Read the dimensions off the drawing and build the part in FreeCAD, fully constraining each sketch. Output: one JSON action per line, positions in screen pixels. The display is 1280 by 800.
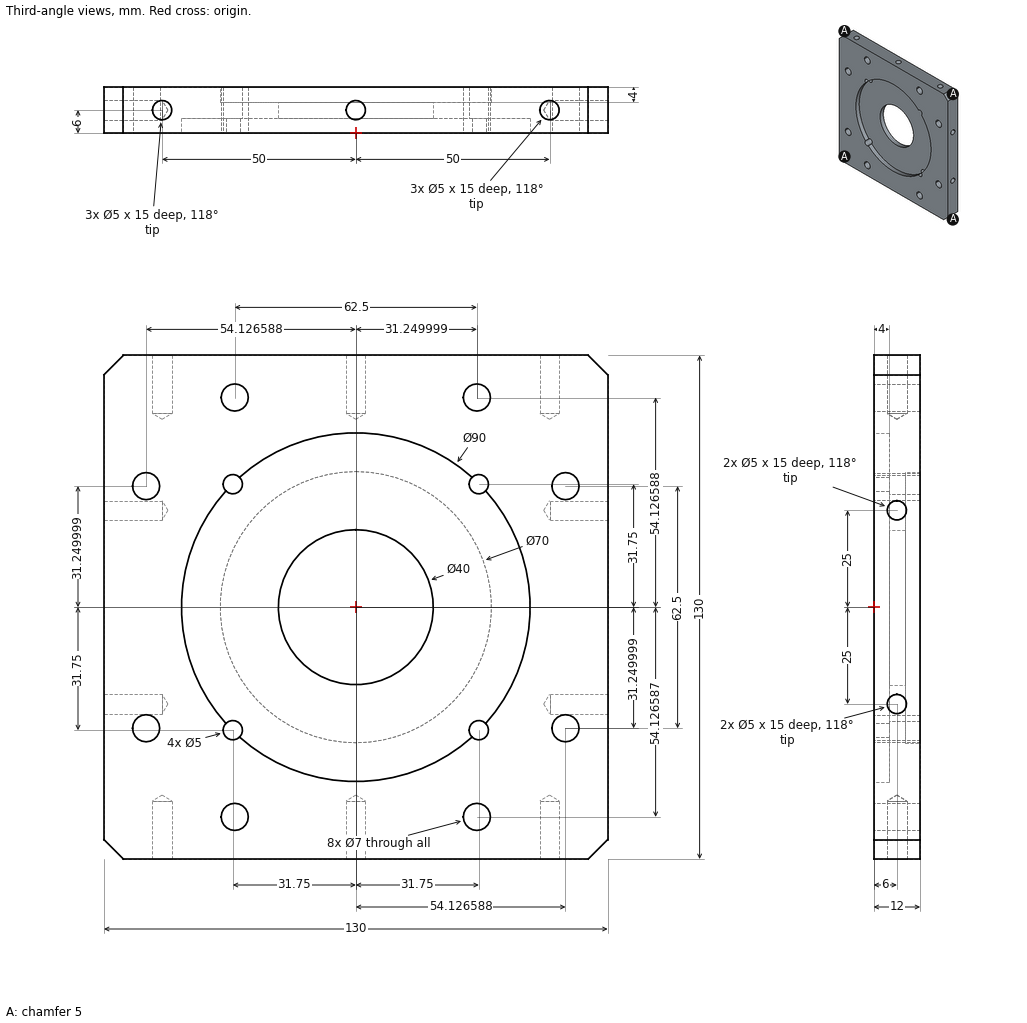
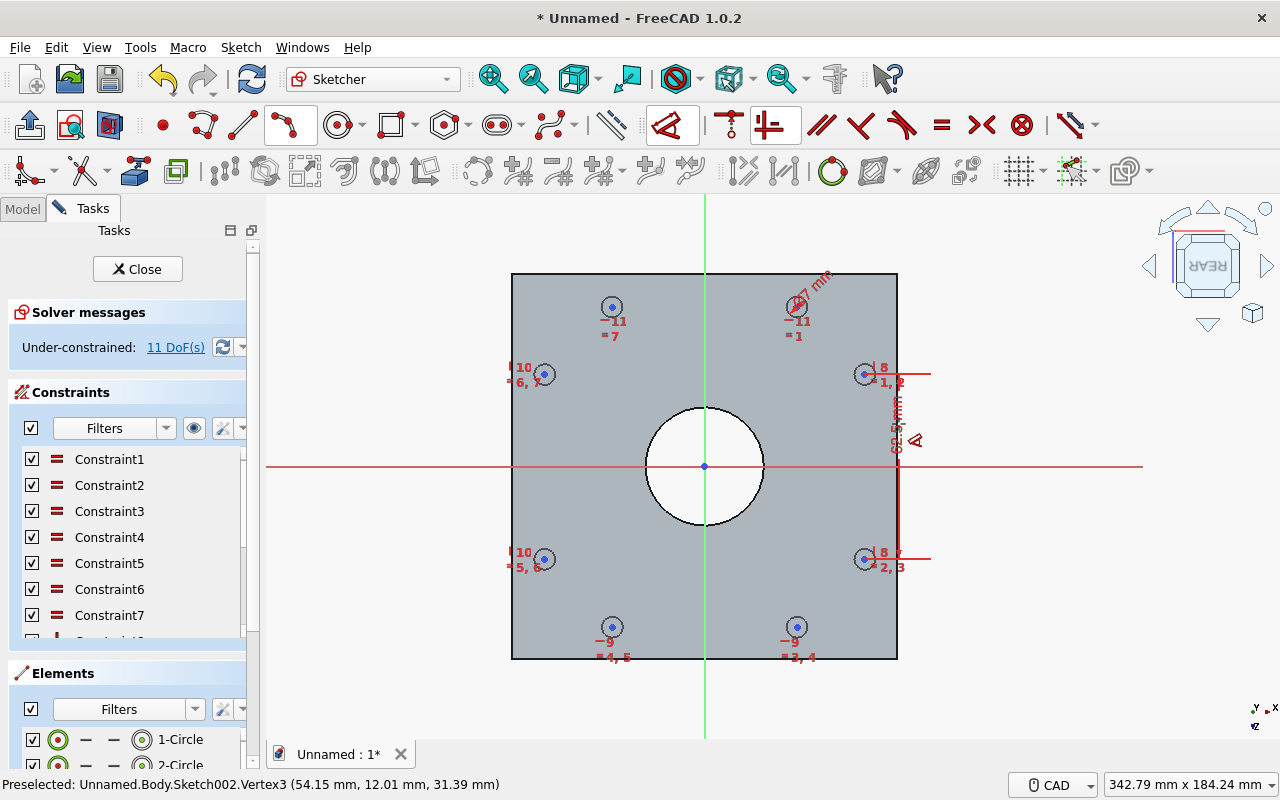
{"action": "left_click", "coordinate": [797, 627]}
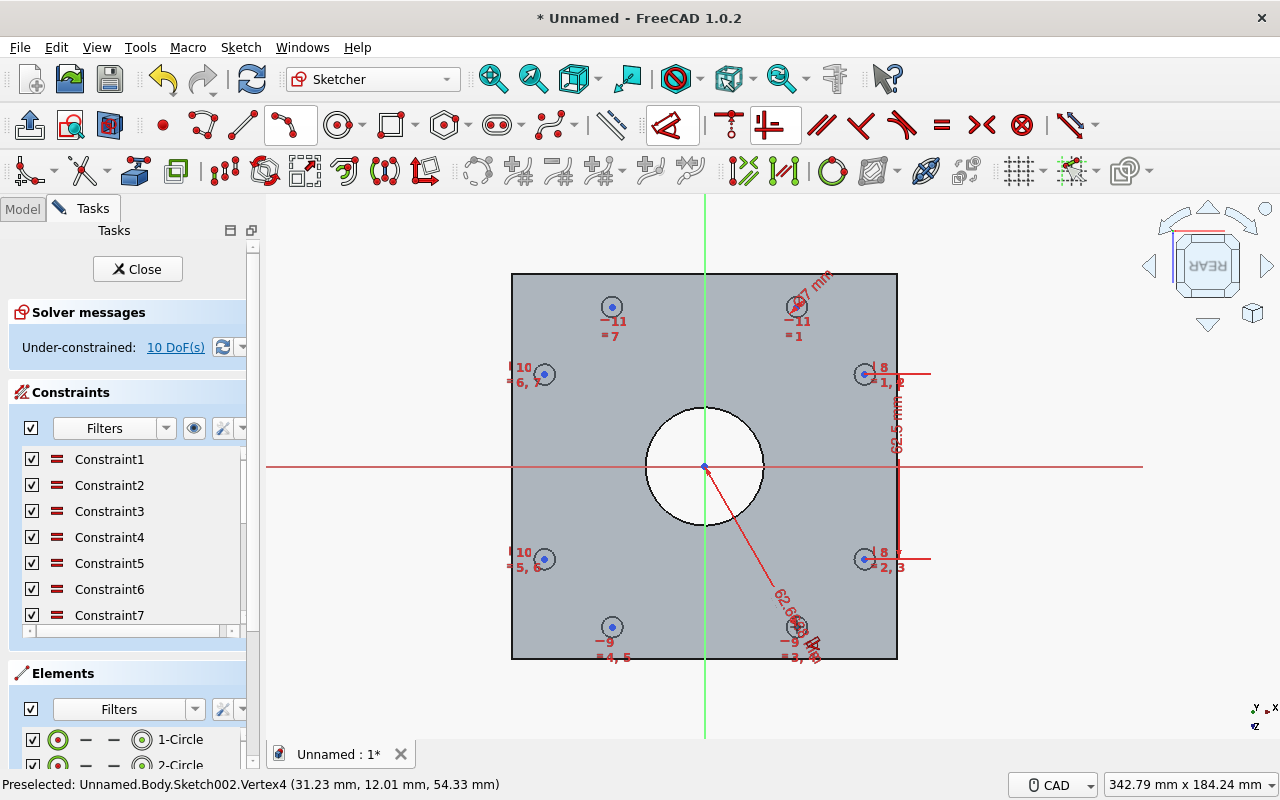
{"action": "left_click", "coordinate": [612, 627]}
{"action": "left_click", "coordinate": [662, 661]}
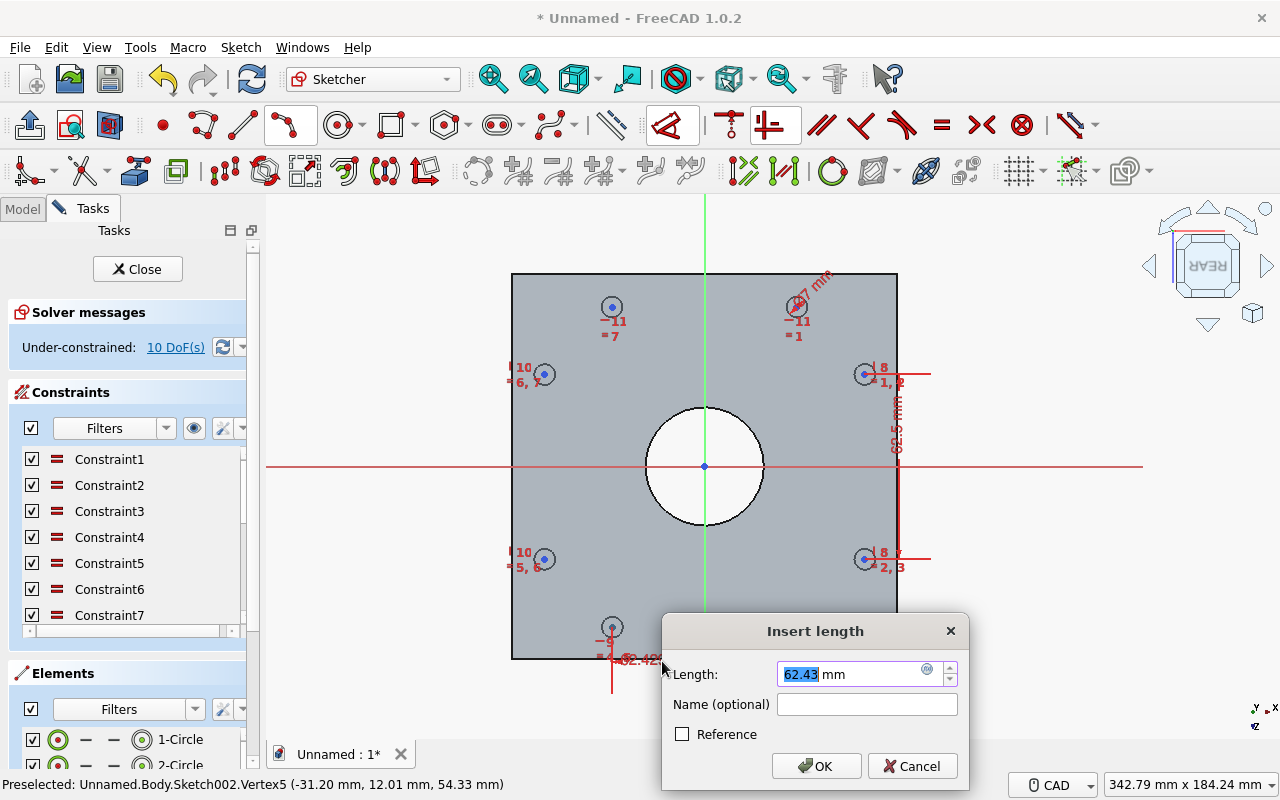
{"action": "type", "text": "62.5"}
{"action": "key", "text": "Return"}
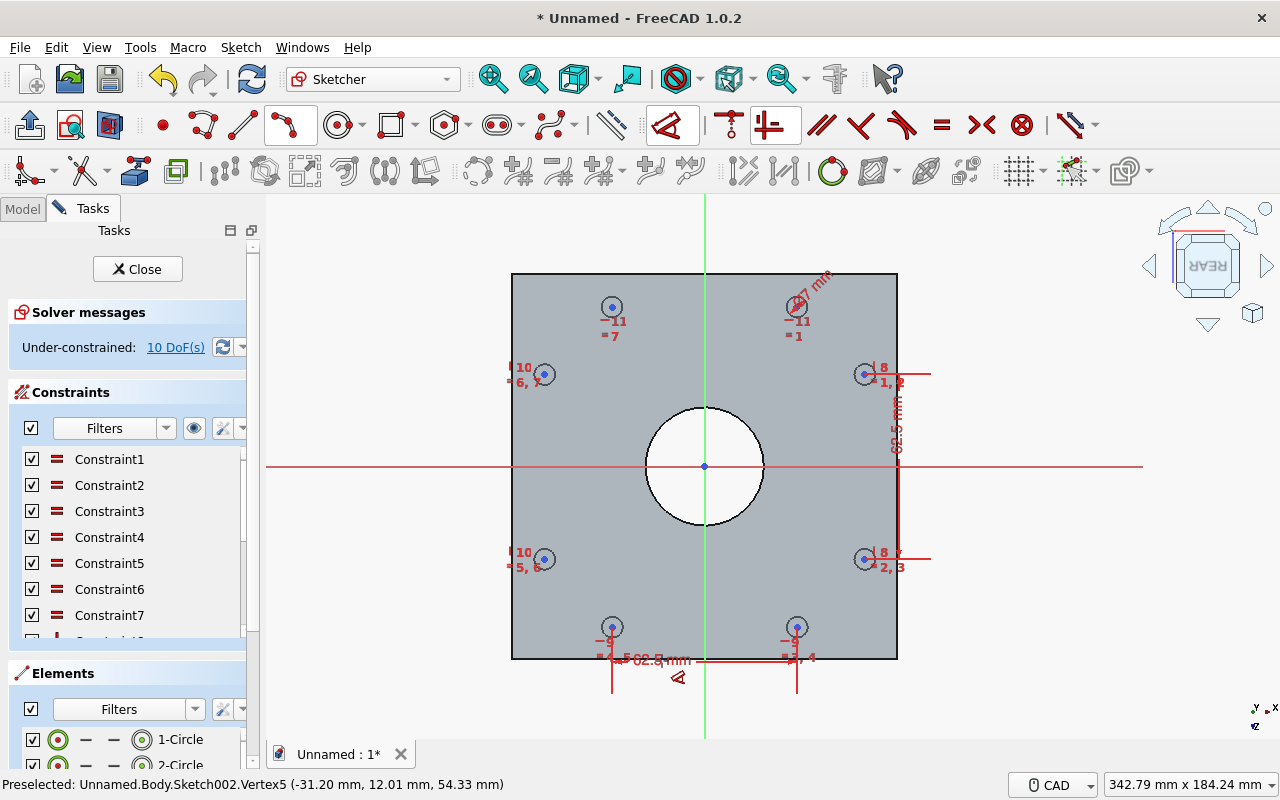
{"action": "left_click", "coordinate": [545, 559]}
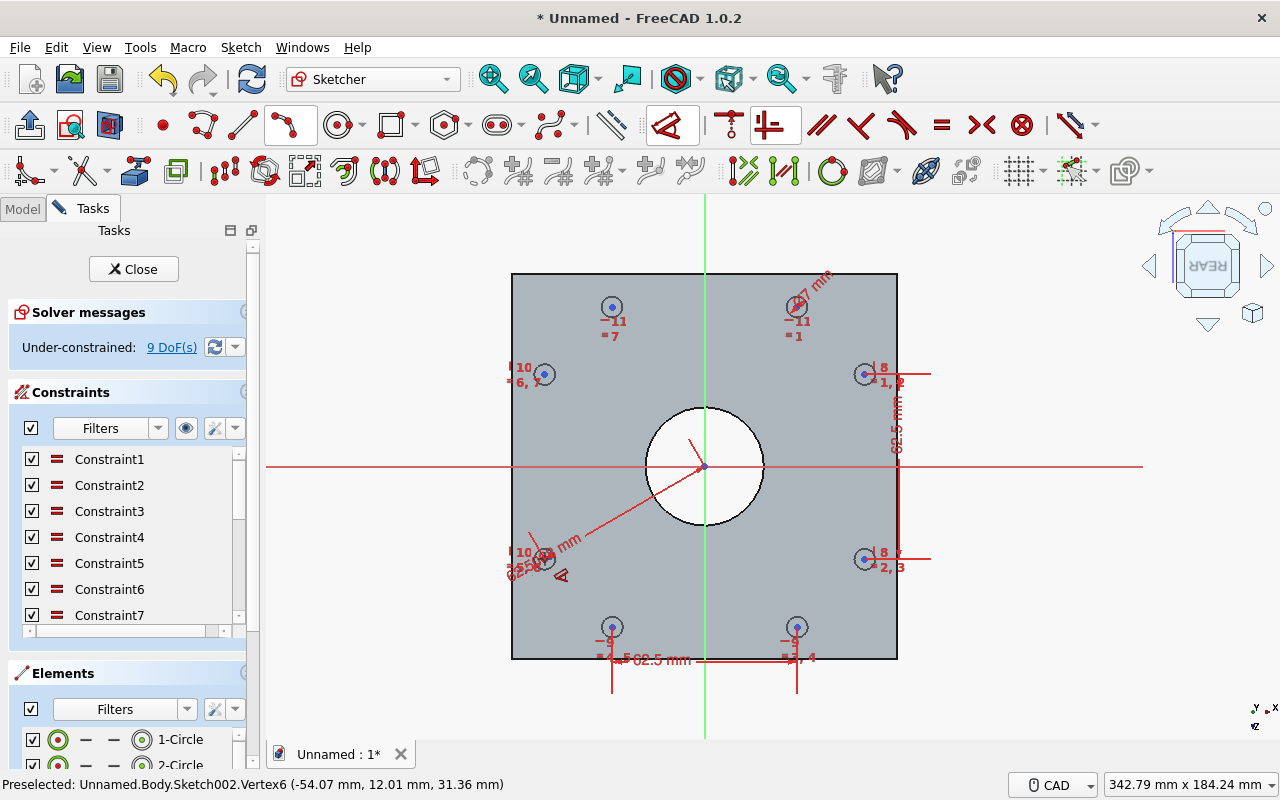
{"action": "left_click", "coordinate": [545, 375]}
{"action": "left_click", "coordinate": [511, 424]}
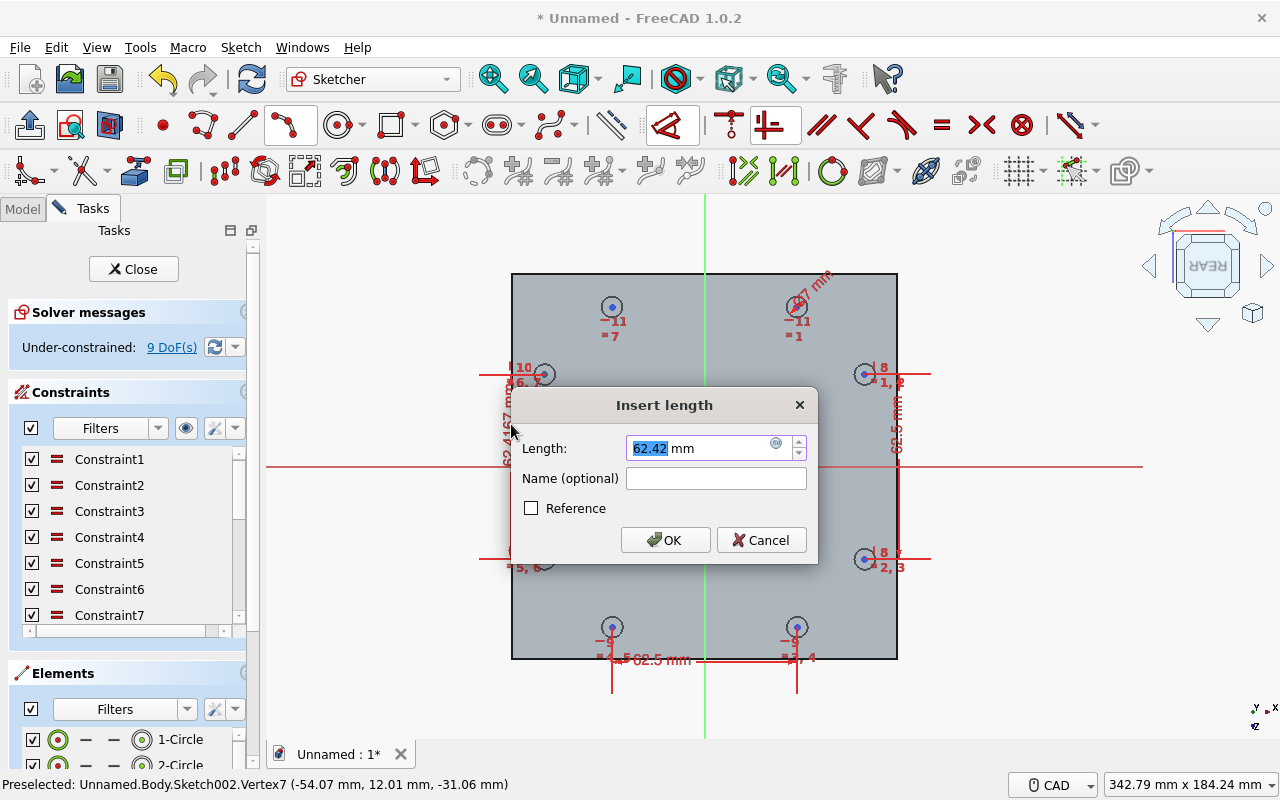
{"action": "type", "text": "62.5"}
{"action": "key", "text": "Return"}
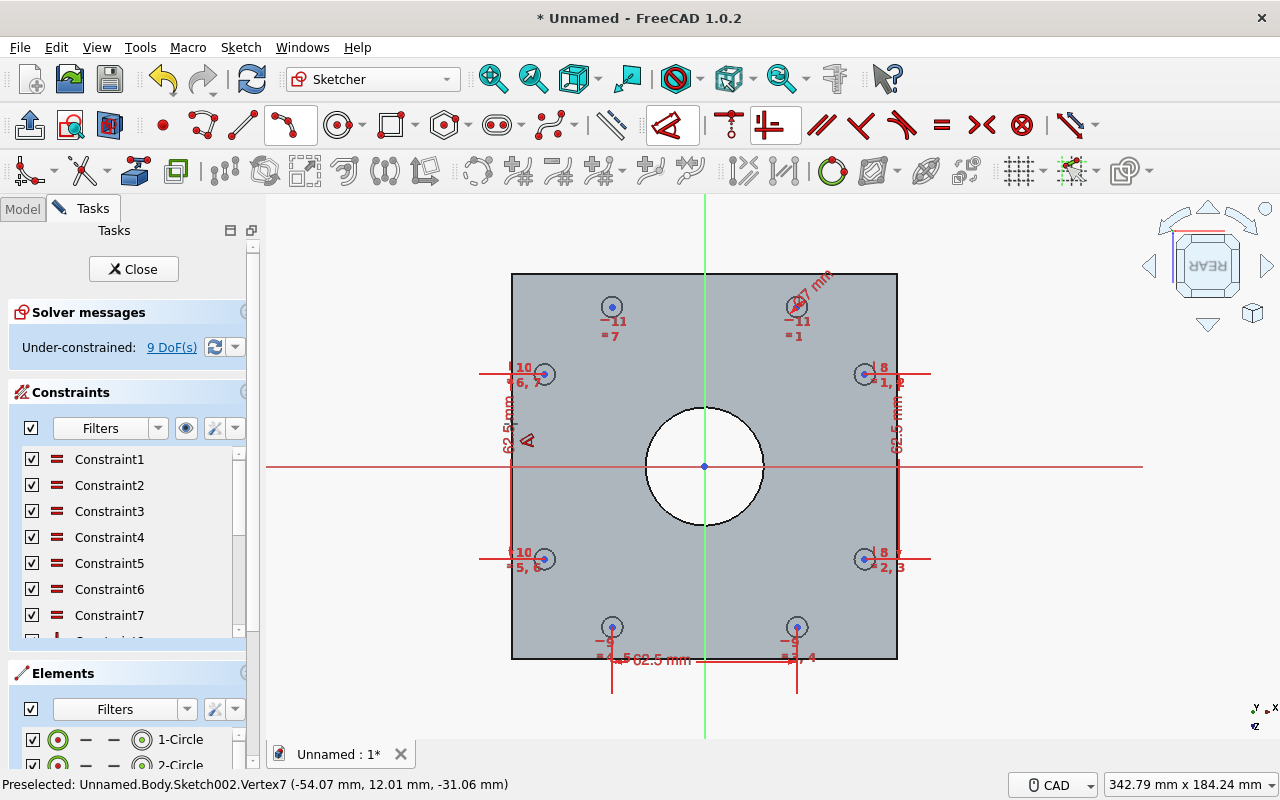
{"action": "left_click", "coordinate": [797, 307]}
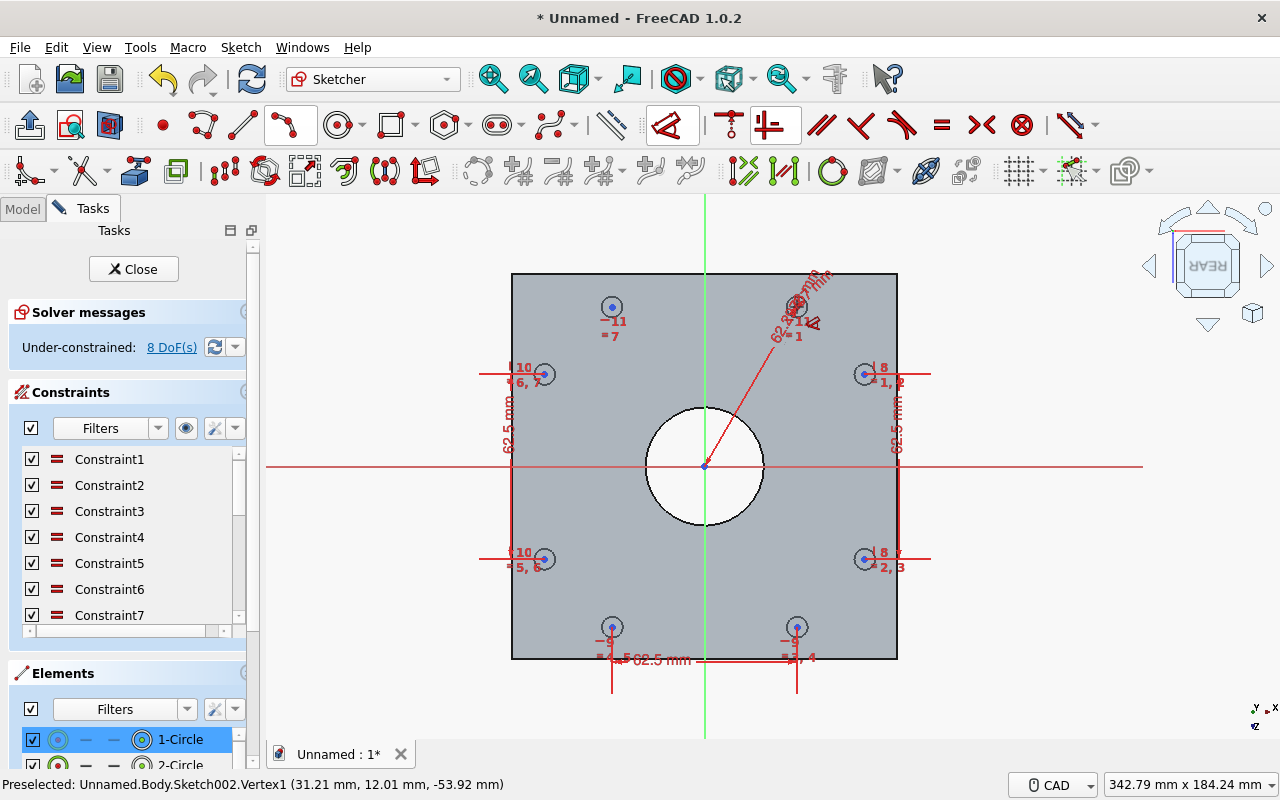
{"action": "left_click", "coordinate": [612, 307]}
{"action": "left_click", "coordinate": [662, 273]}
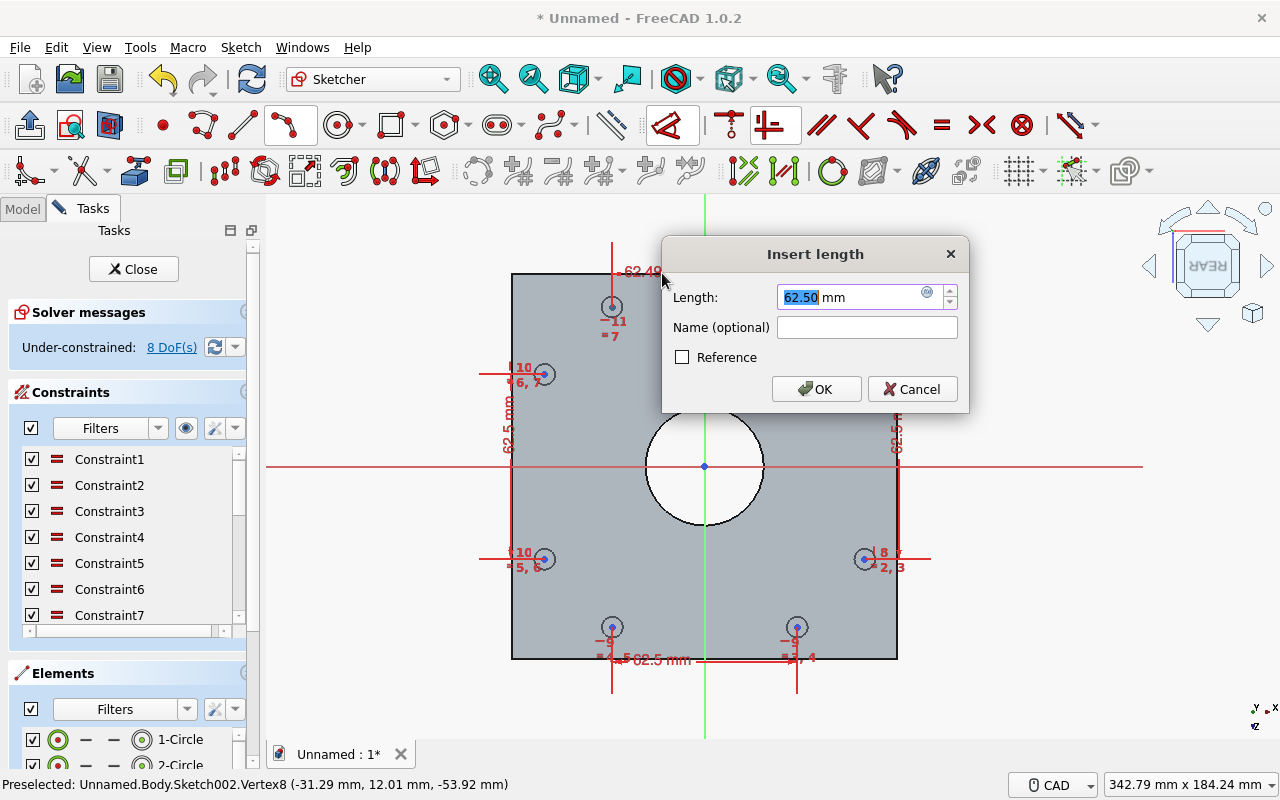
{"action": "type", "text": "62.5"}
{"action": "key", "text": "Return"}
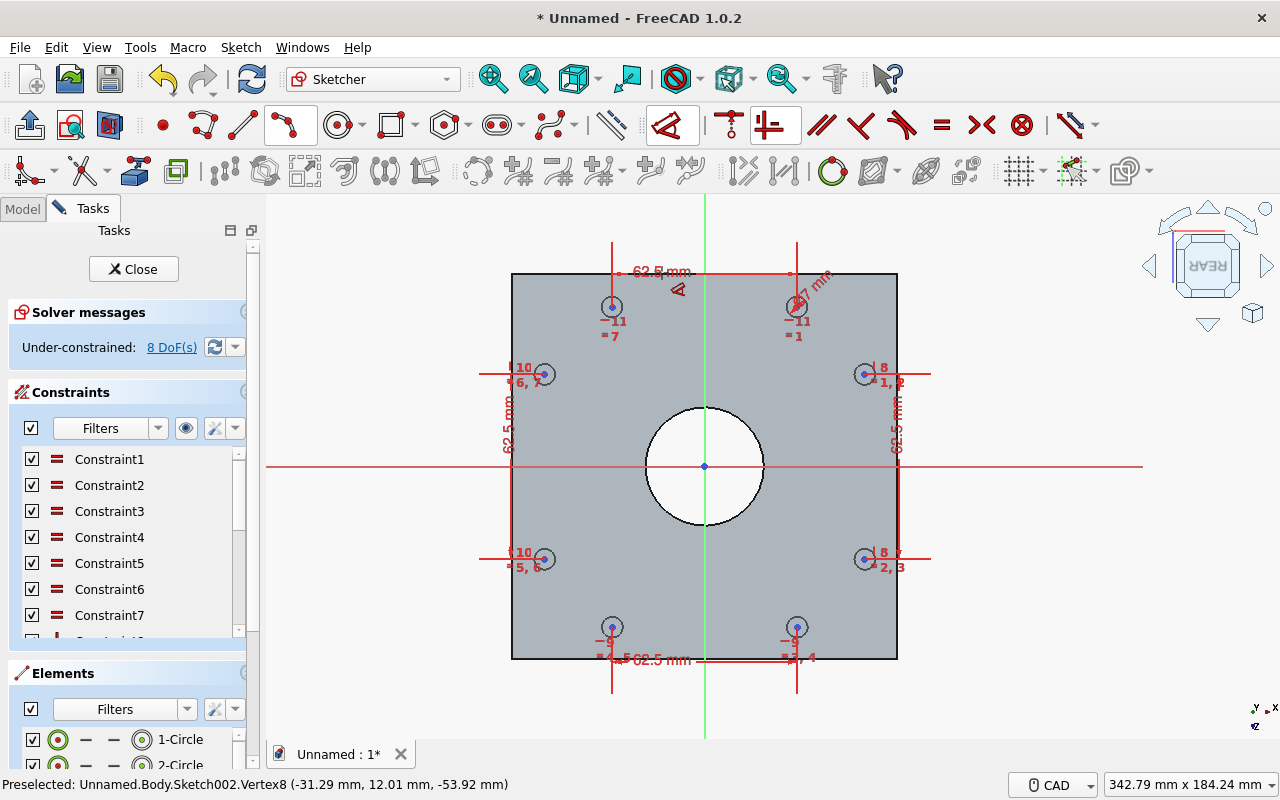
{"action": "left_click", "coordinate": [797, 307]}
{"action": "left_click", "coordinate": [751, 500]}